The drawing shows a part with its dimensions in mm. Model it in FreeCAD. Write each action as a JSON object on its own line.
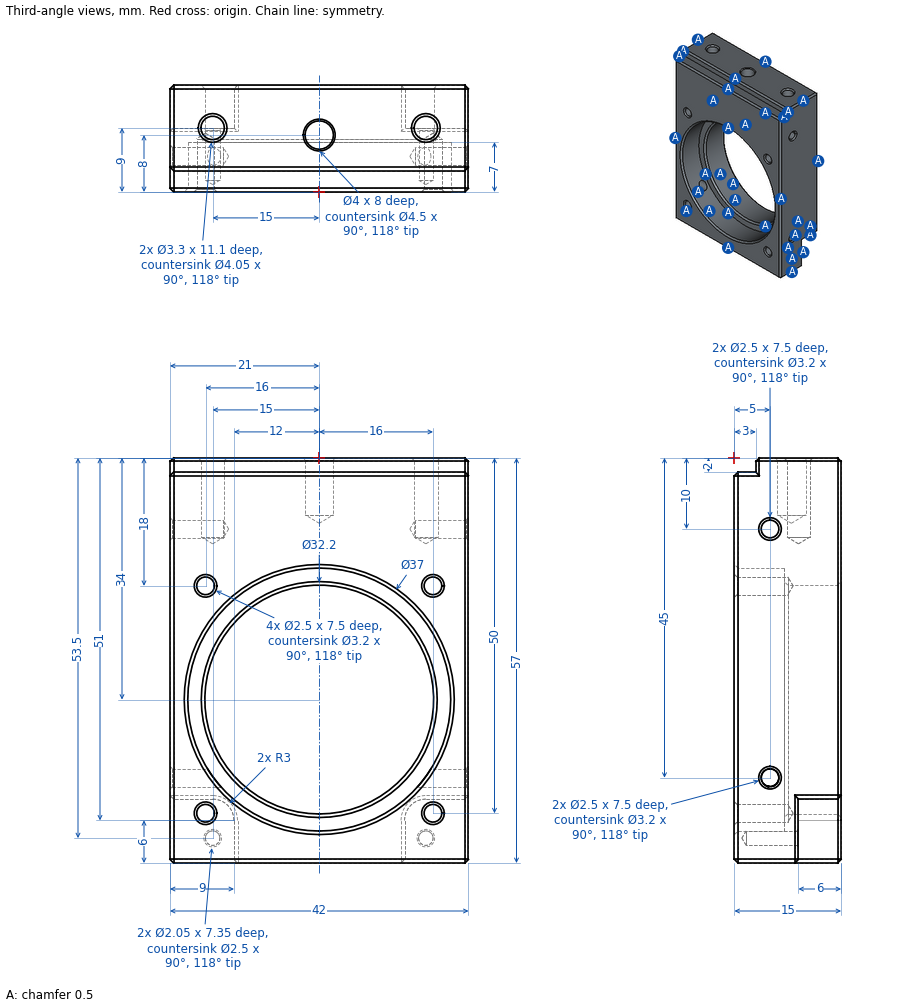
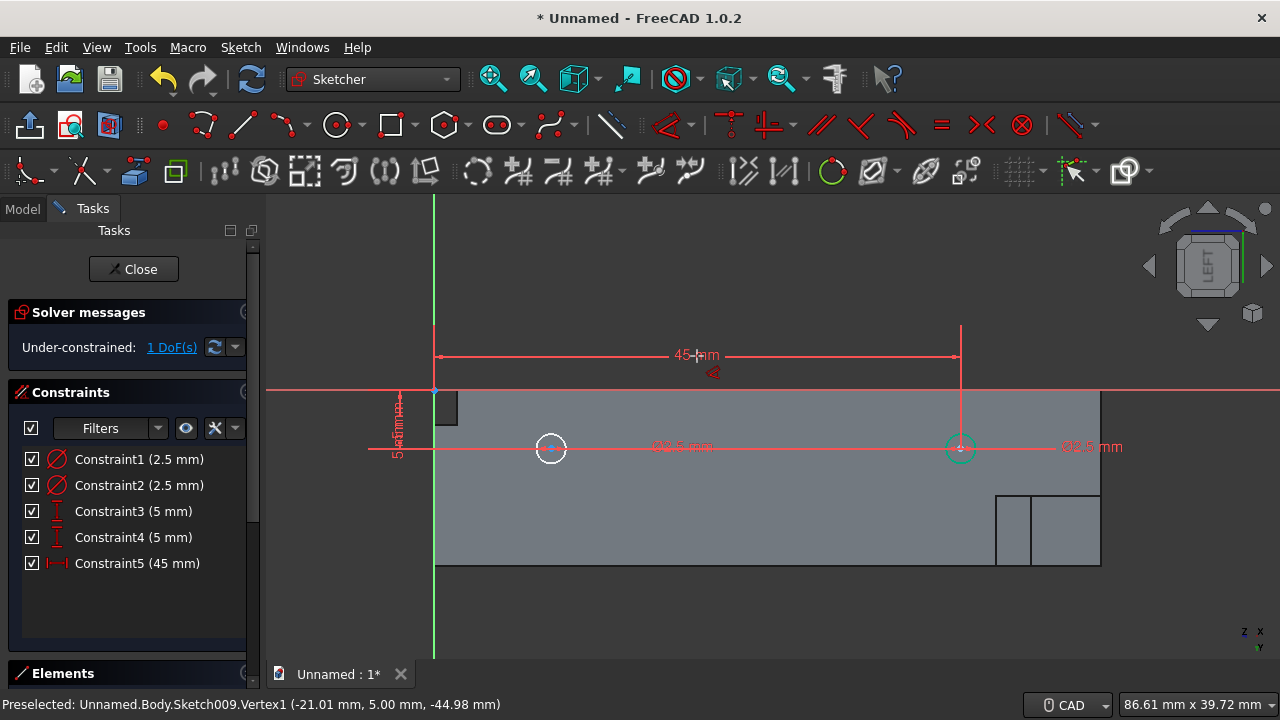
{"action": "left_click", "coordinate": [551, 449]}
{"action": "left_click", "coordinate": [493, 356]}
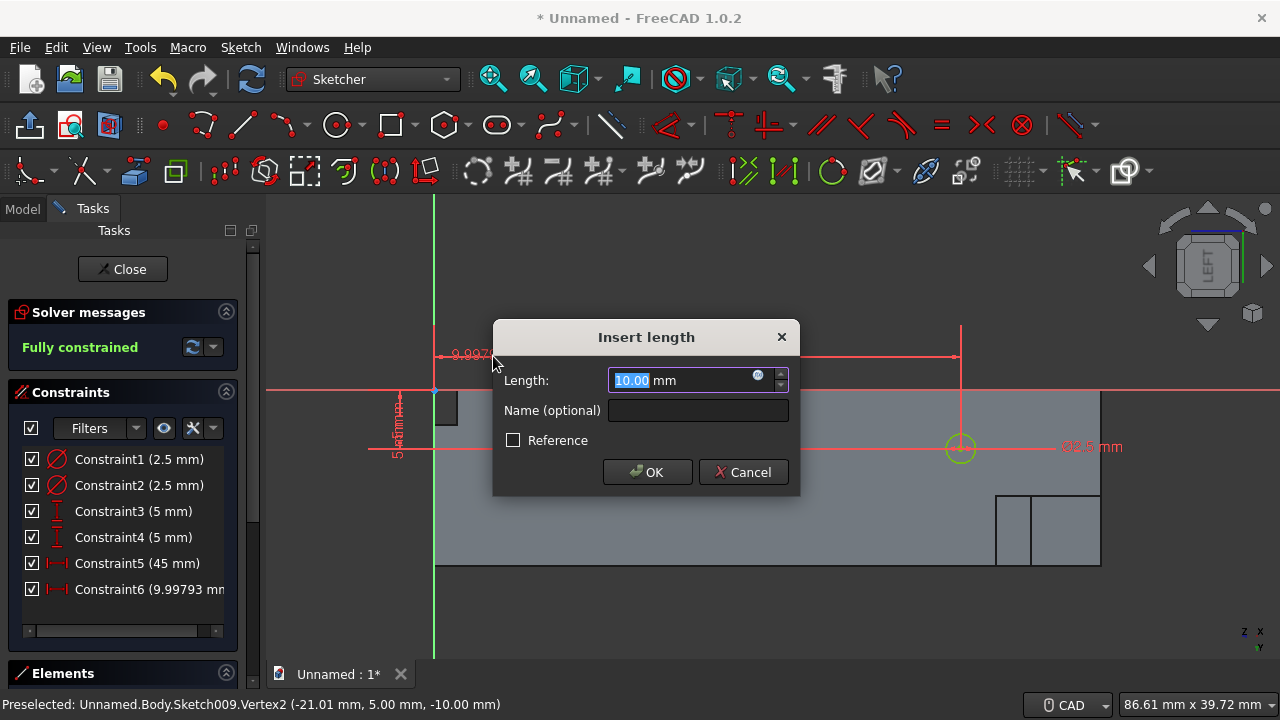
{"action": "type", "text": "10"}
{"action": "key", "text": "Return"}
{"action": "key", "text": "Escape"}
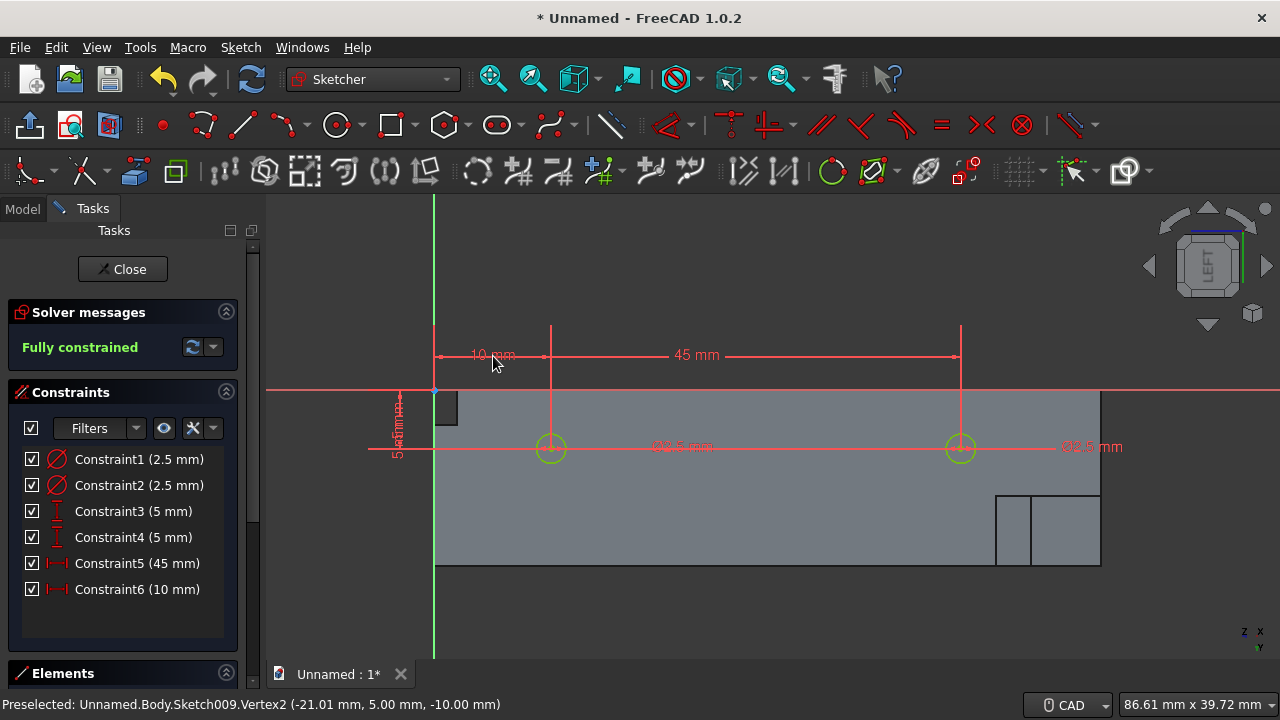
{"action": "left_click", "coordinate": [123, 269]}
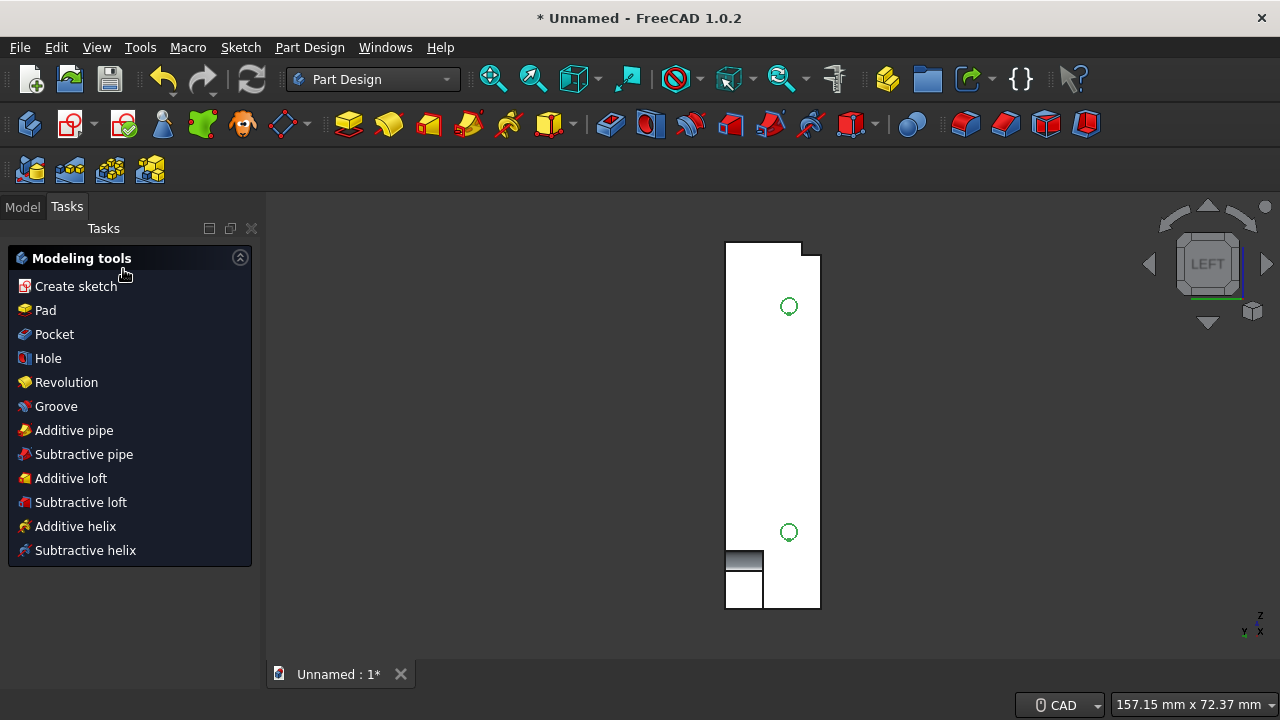
{"action": "left_click", "coordinate": [652, 124]}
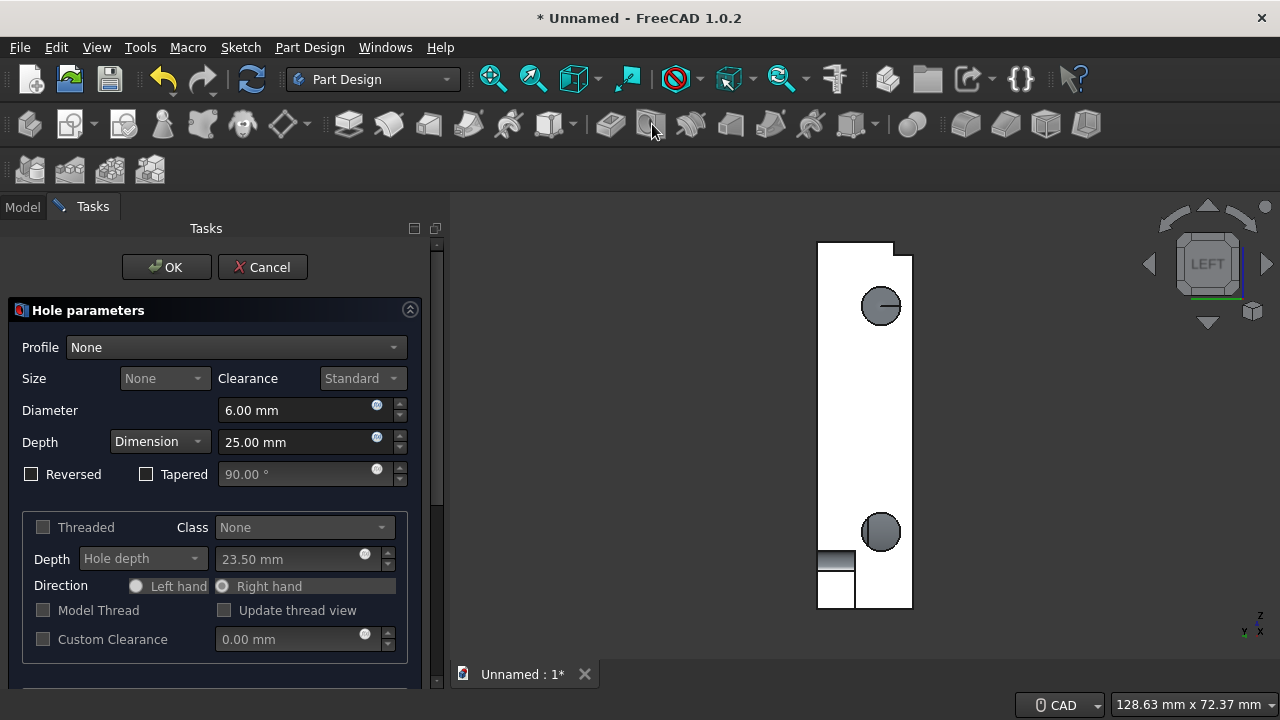
{"action": "triple_click", "coordinate": [305, 410]}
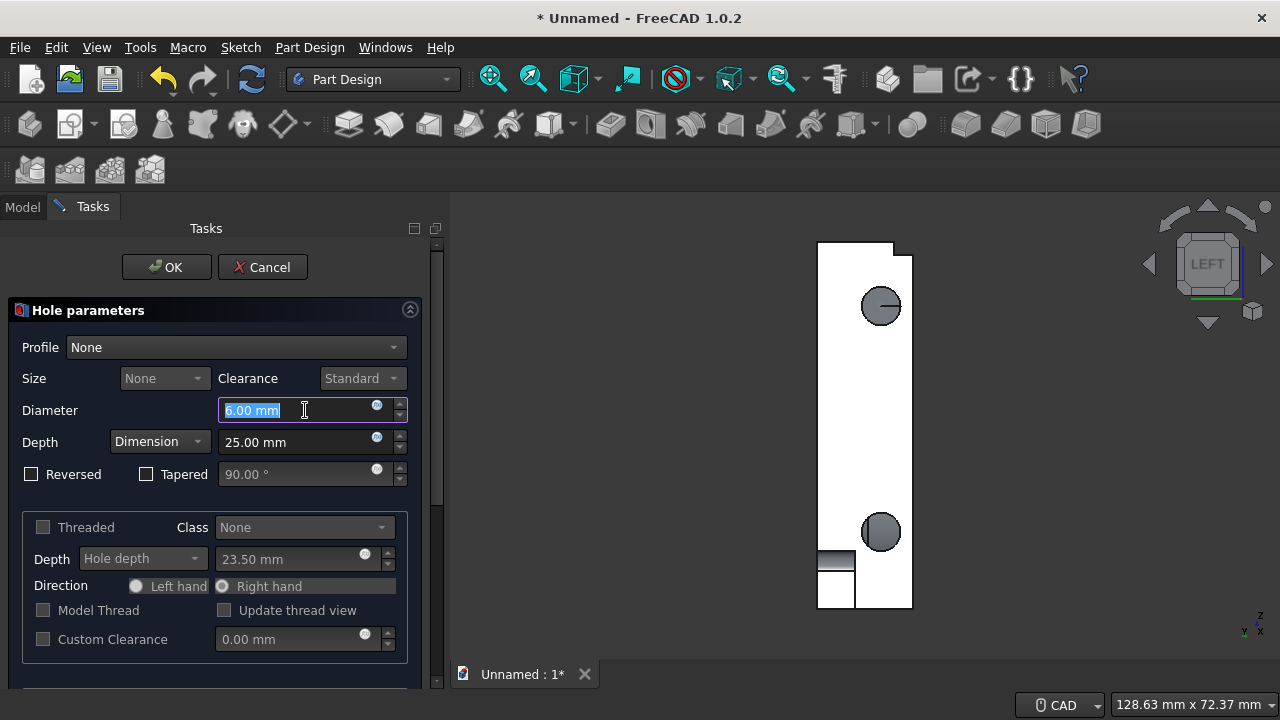
{"action": "type", "text": "2.5"}
{"action": "key", "text": "Tab"}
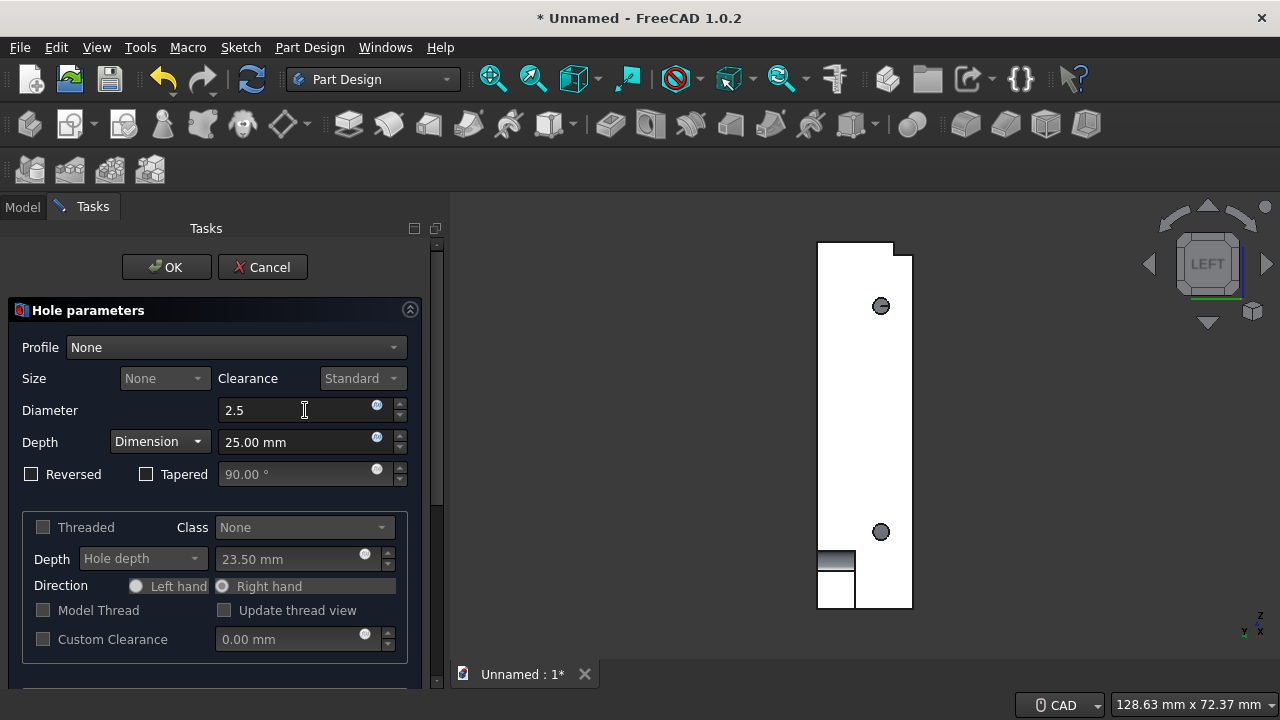
{"action": "triple_click", "coordinate": [305, 442]}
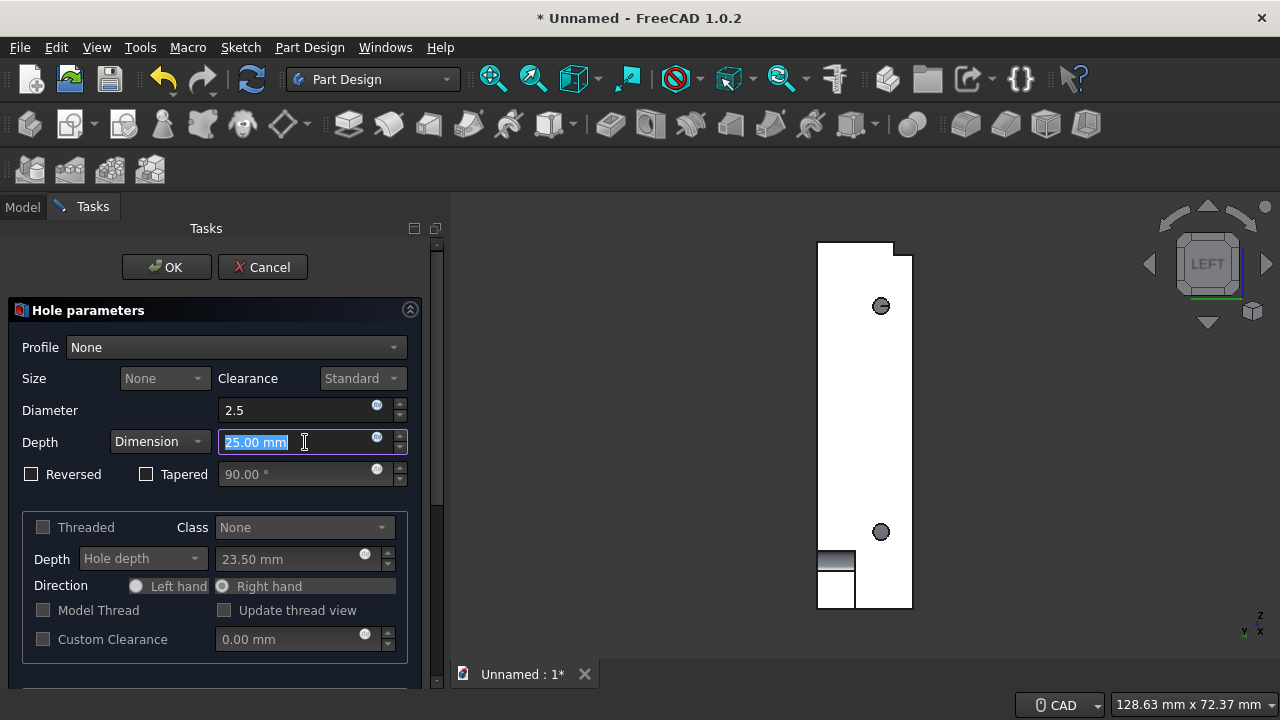
{"action": "type", "text": "7.5"}
{"action": "key", "text": "Tab"}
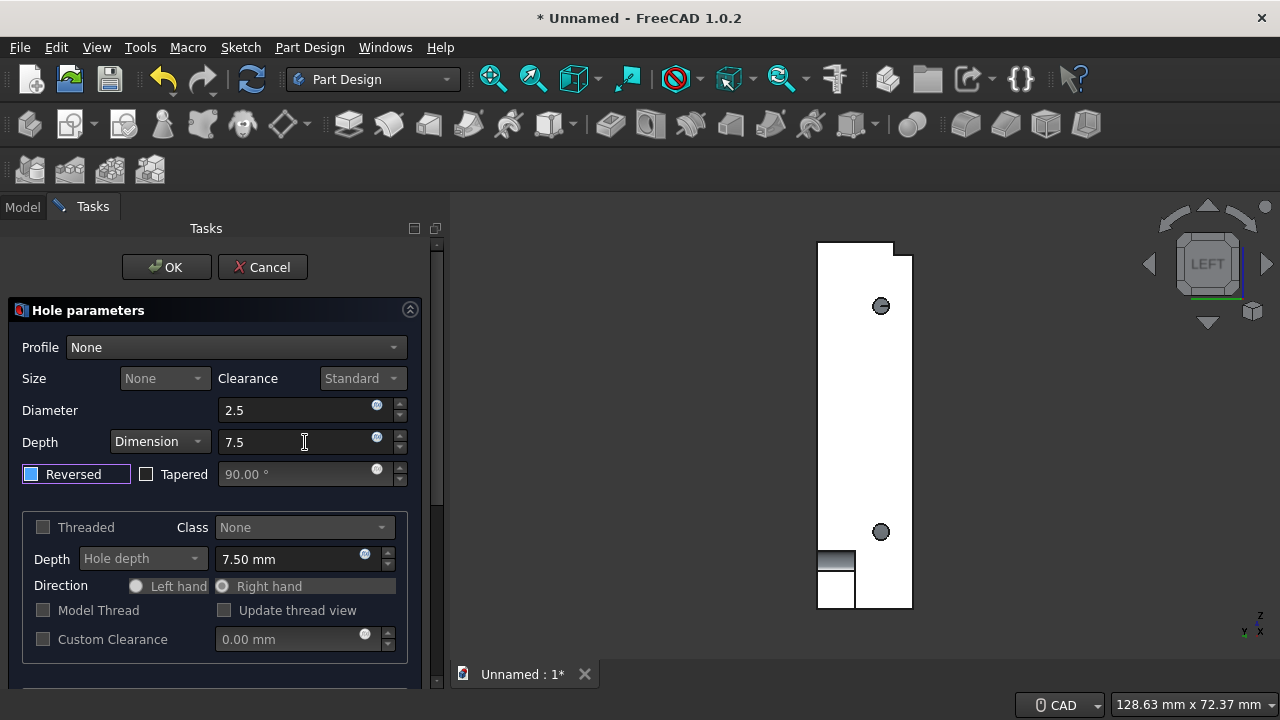
{"action": "scroll", "coordinate": [437, 463], "scroll_direction": "down", "scroll_amount": 2}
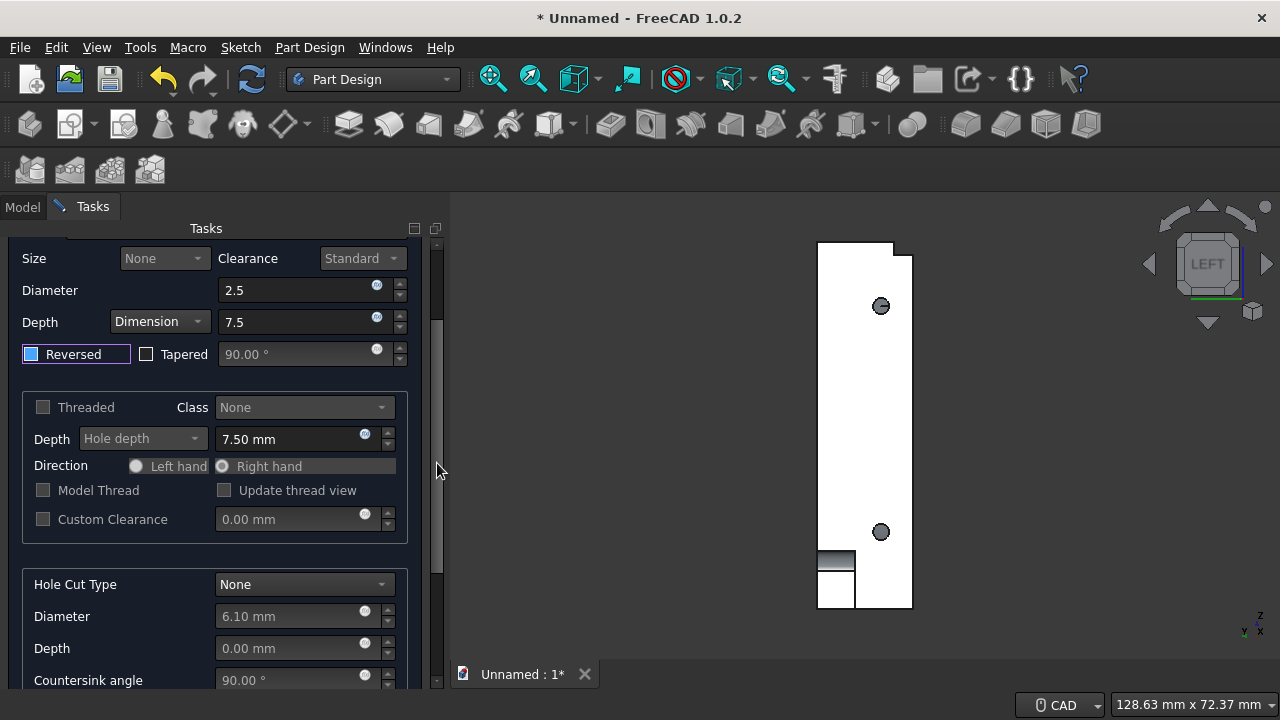
{"action": "left_click", "coordinate": [306, 584]}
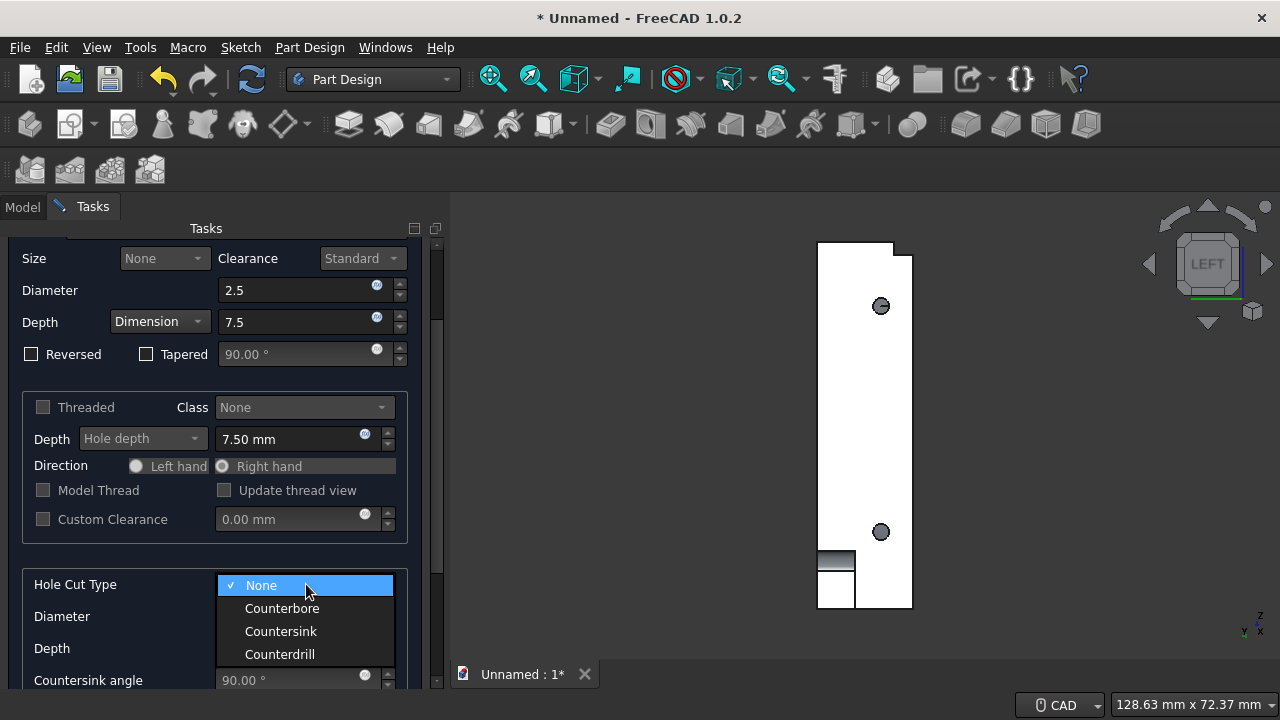
{"action": "left_click", "coordinate": [304, 632]}